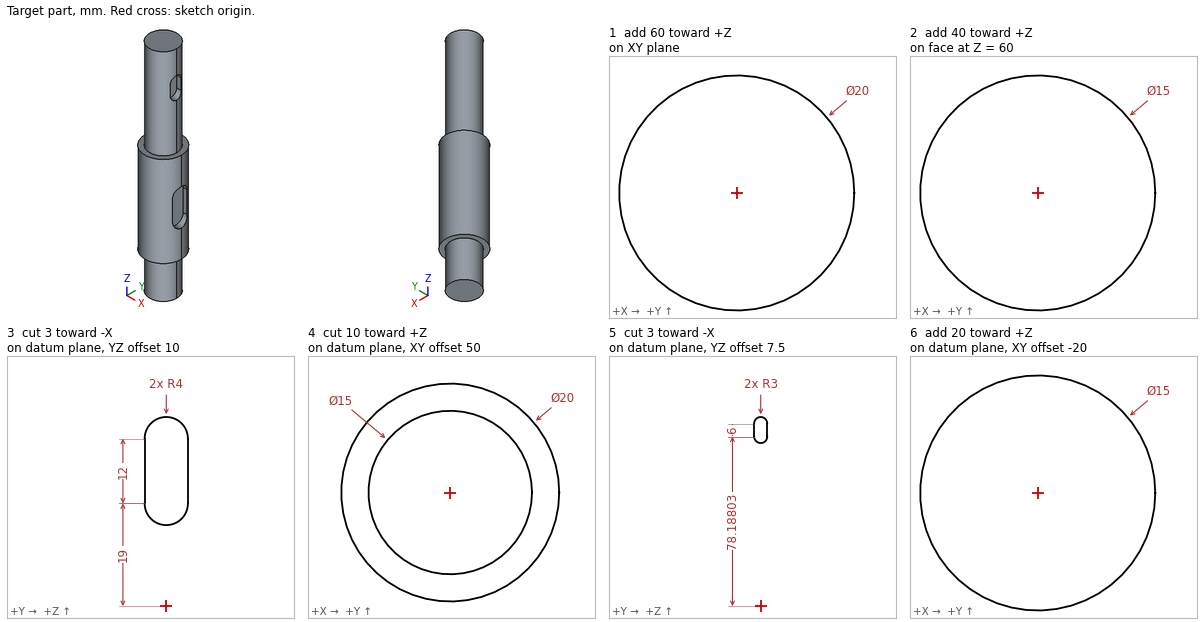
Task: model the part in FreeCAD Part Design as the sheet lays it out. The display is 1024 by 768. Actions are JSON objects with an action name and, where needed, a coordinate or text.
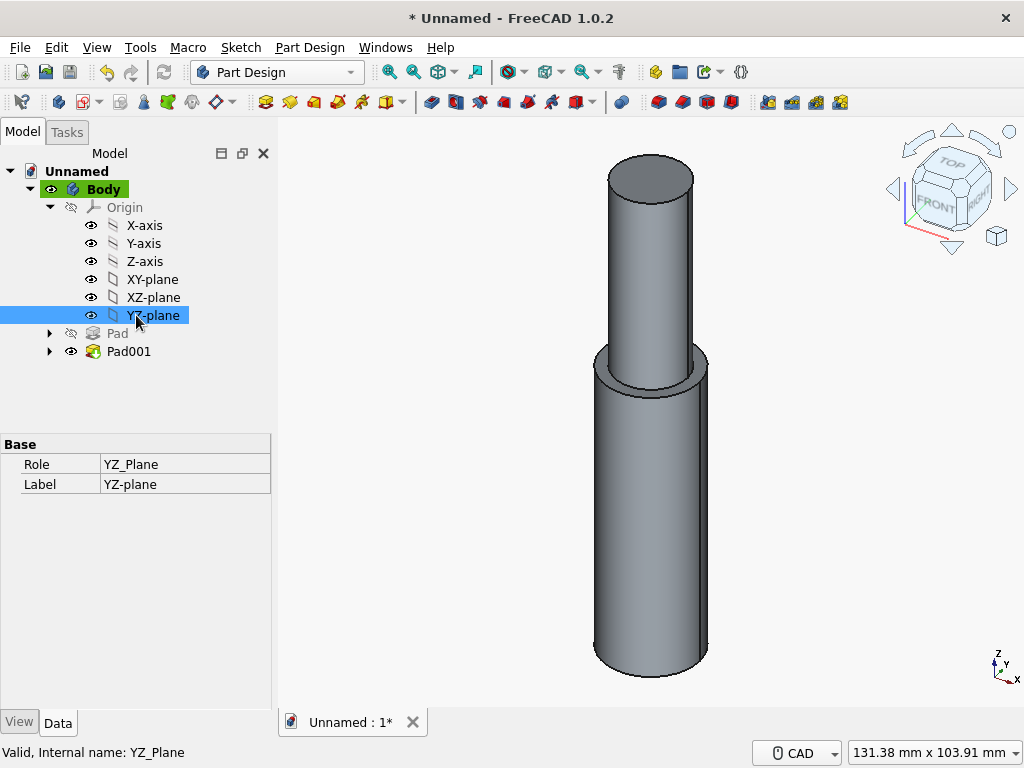
{"action": "left_click", "coordinate": [216, 102]}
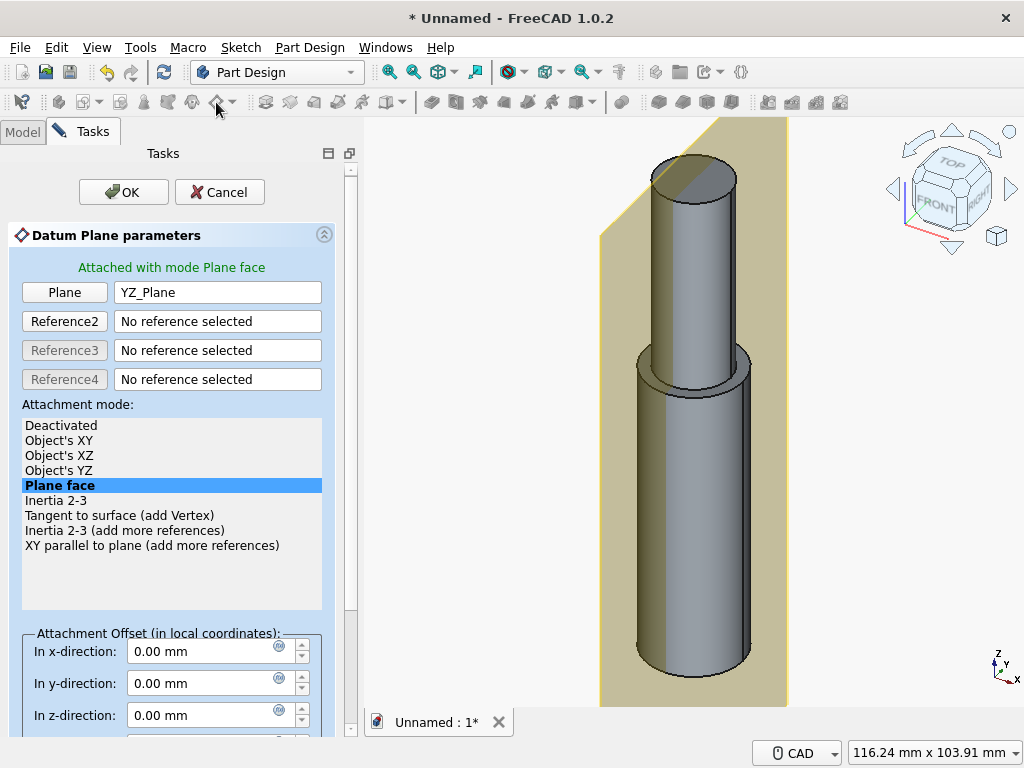
{"action": "triple_click", "coordinate": [210, 715]}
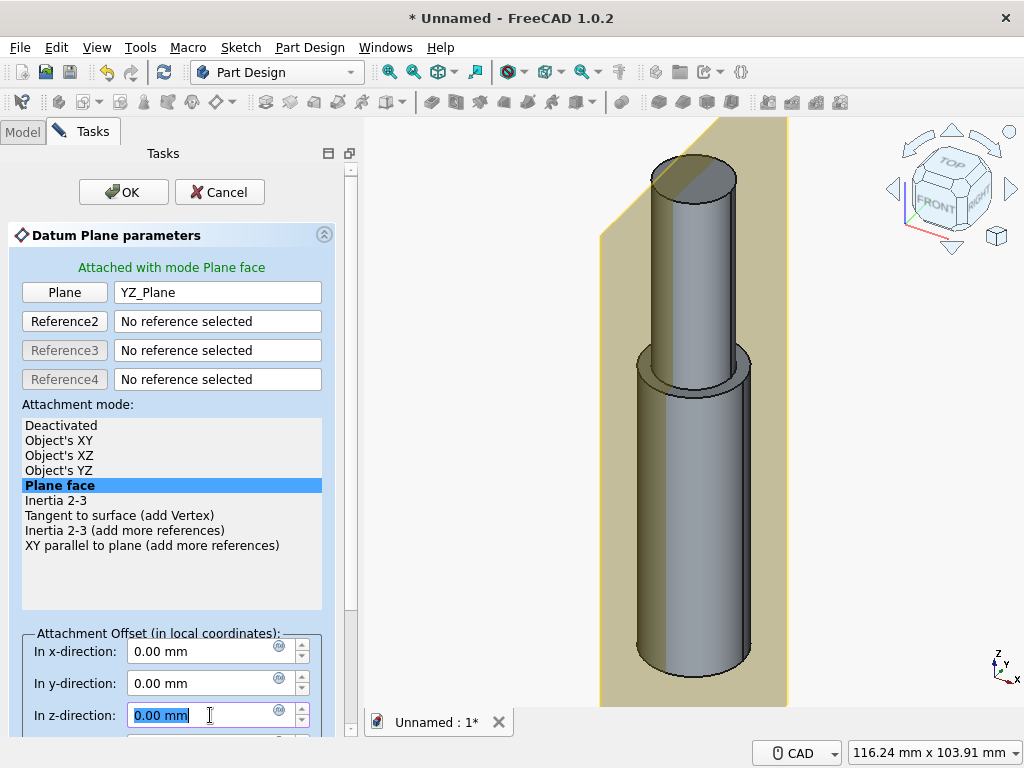
{"action": "type", "text": "10"}
{"action": "key", "text": "Tab"}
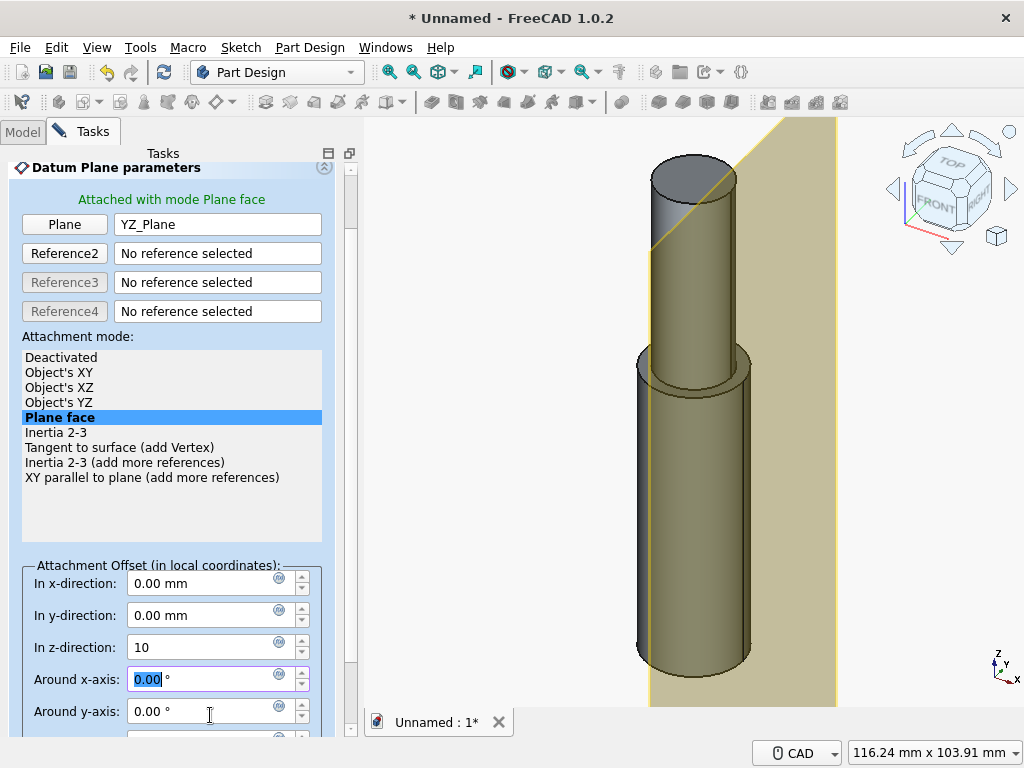
{"action": "scroll", "coordinate": [351, 450], "scroll_direction": "up", "scroll_amount": 2}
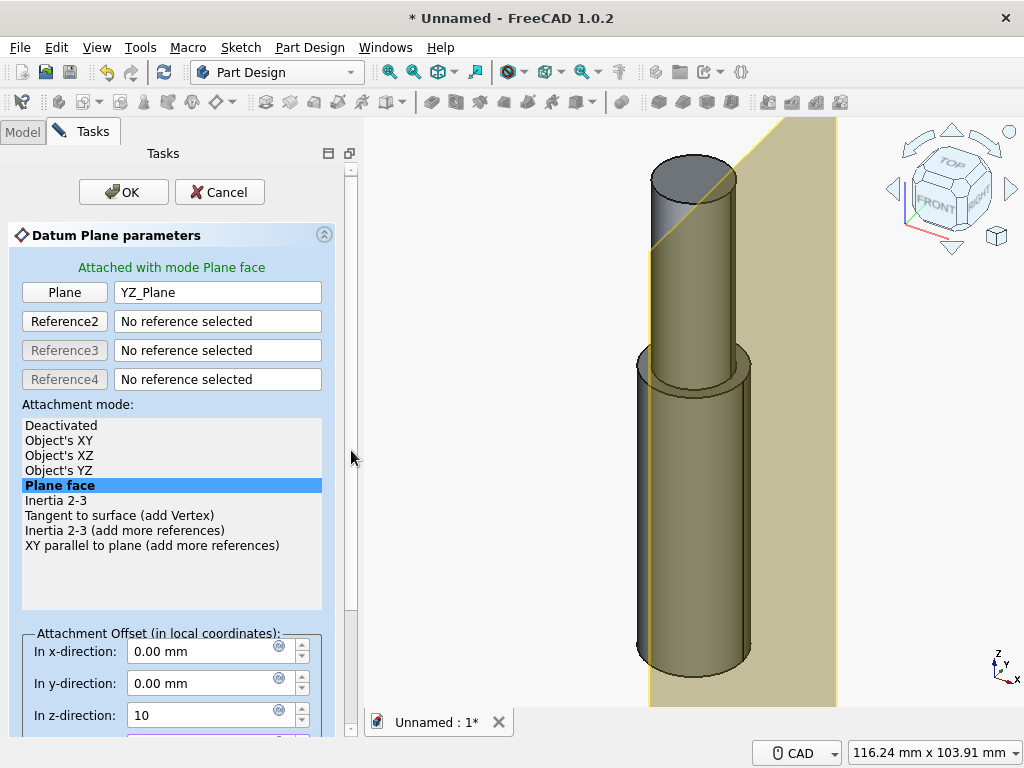
{"action": "left_click", "coordinate": [124, 192]}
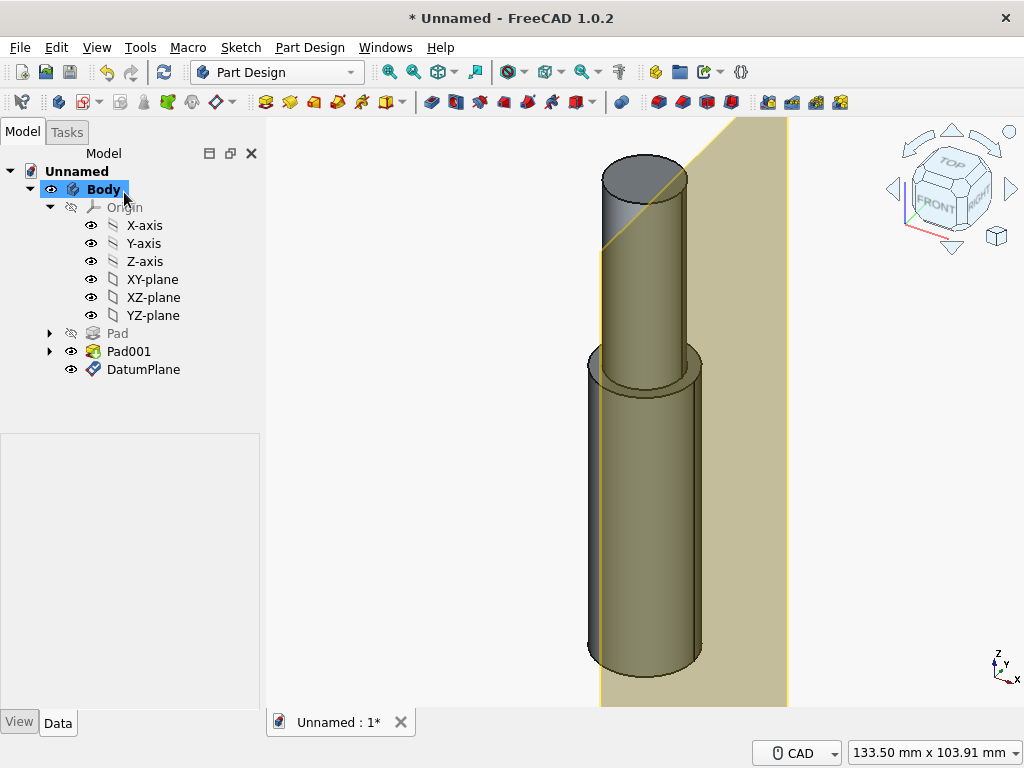
{"action": "left_click", "coordinate": [116, 369]}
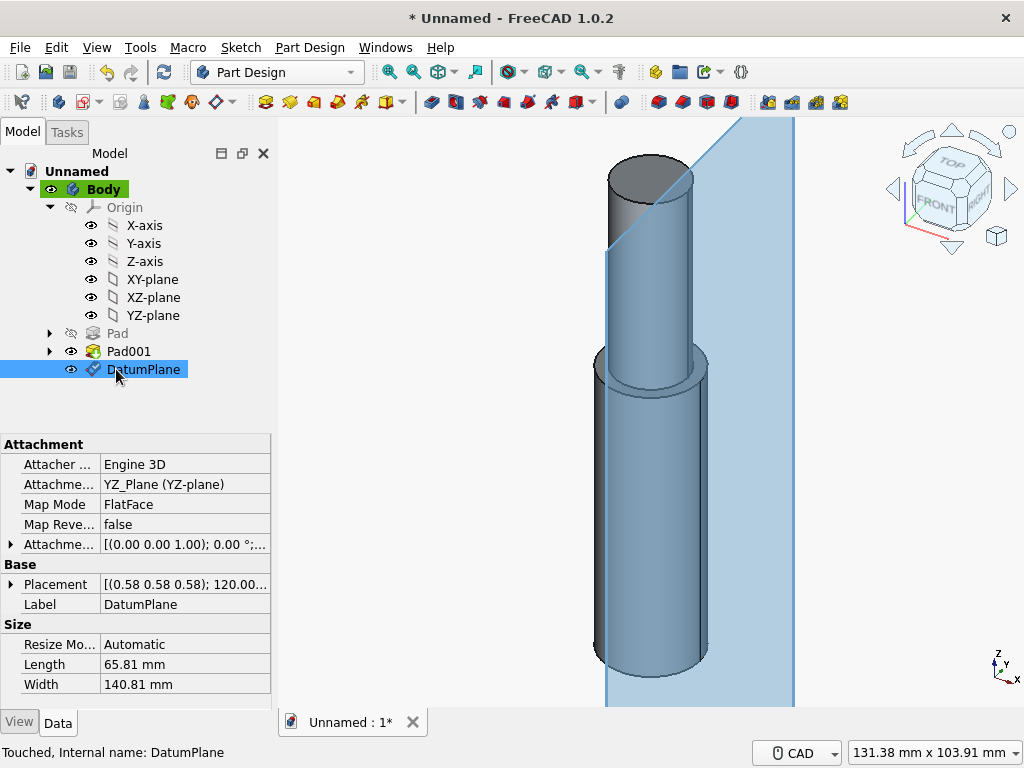
{"action": "left_click", "coordinate": [84, 102]}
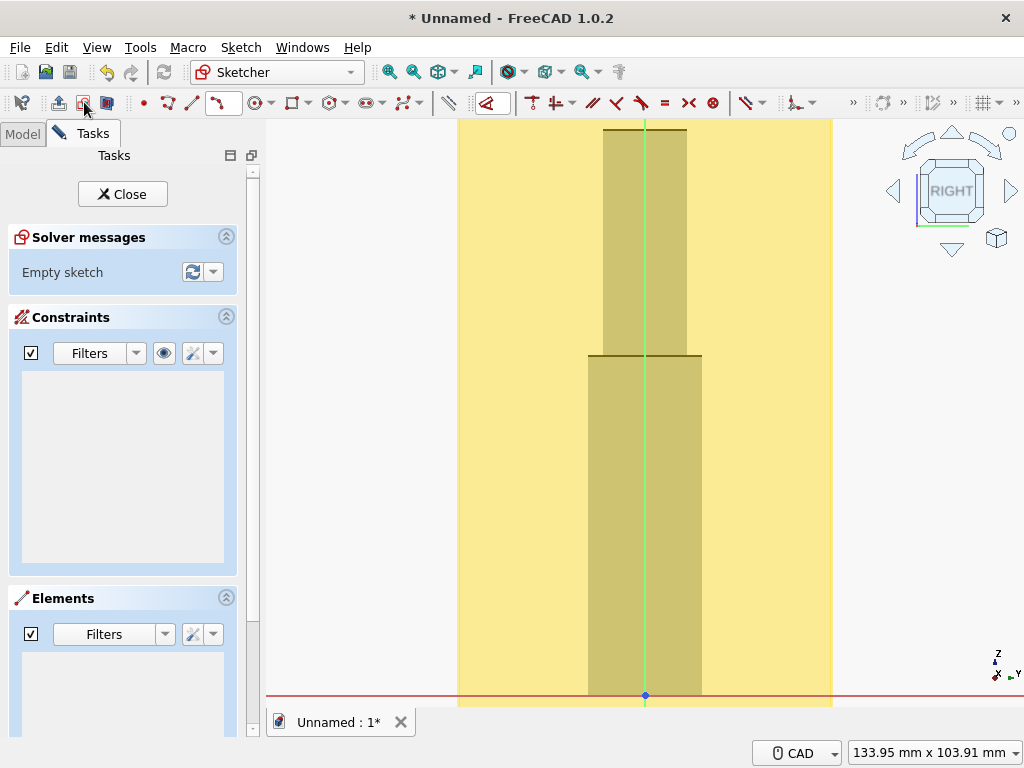
{"action": "scroll", "coordinate": [576, 413], "scroll_direction": "down", "scroll_amount": 5}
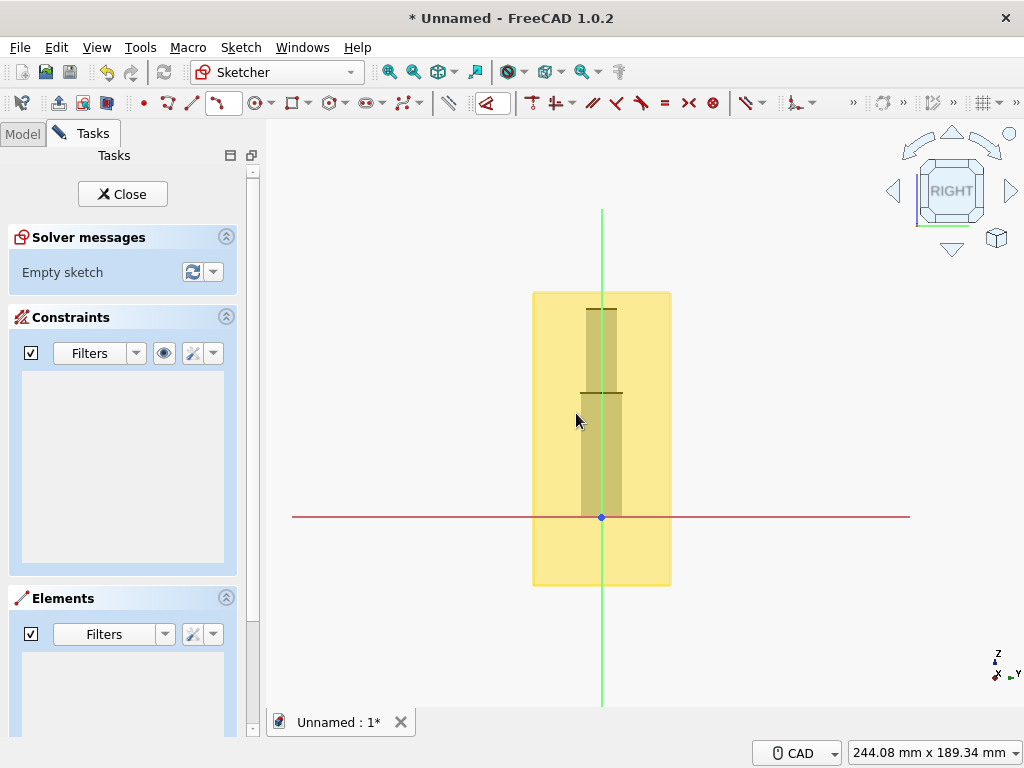
{"action": "scroll", "coordinate": [608, 498], "scroll_direction": "up", "scroll_amount": 8}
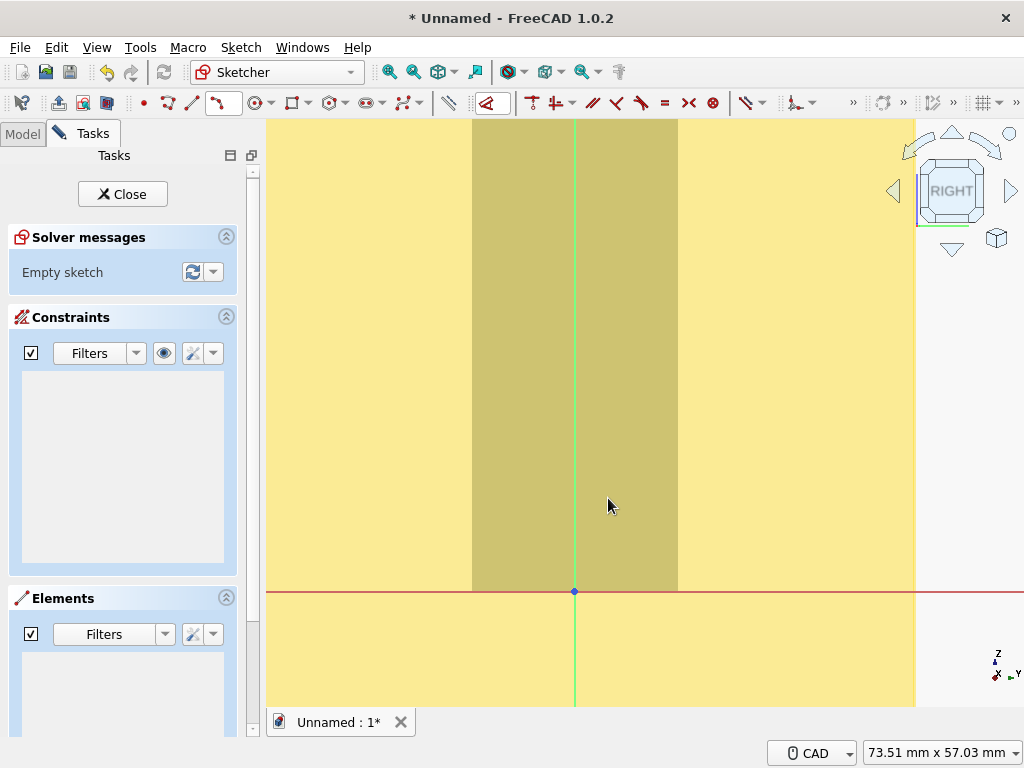
{"action": "left_click", "coordinate": [366, 104]}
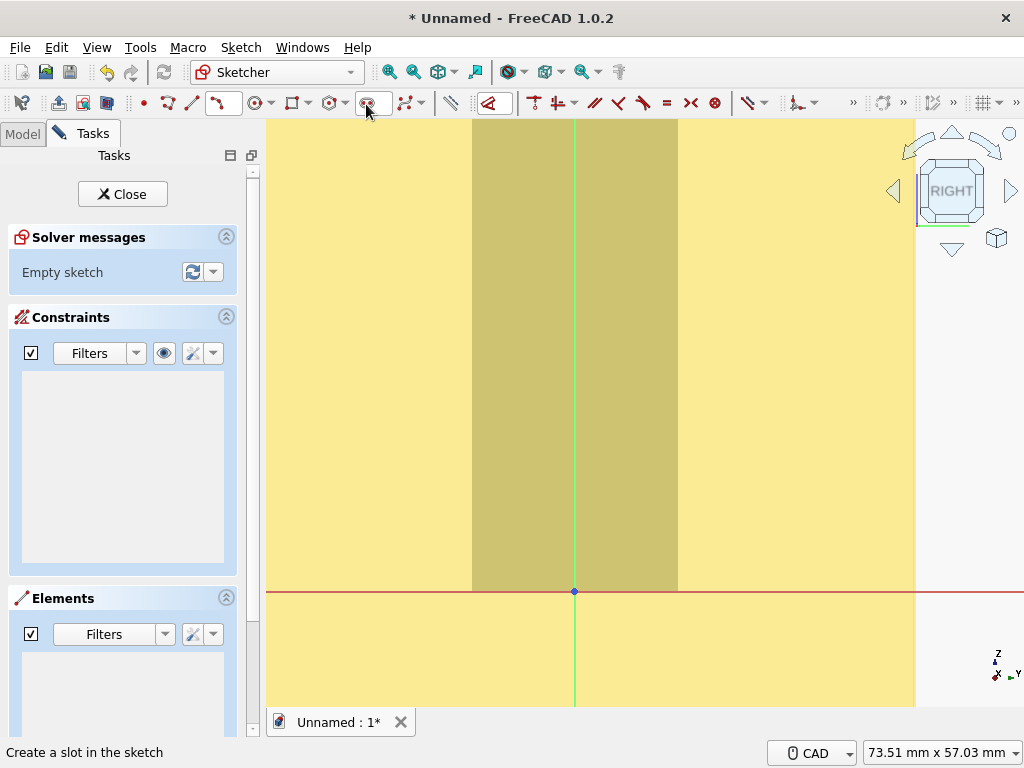
{"action": "left_click", "coordinate": [575, 396]}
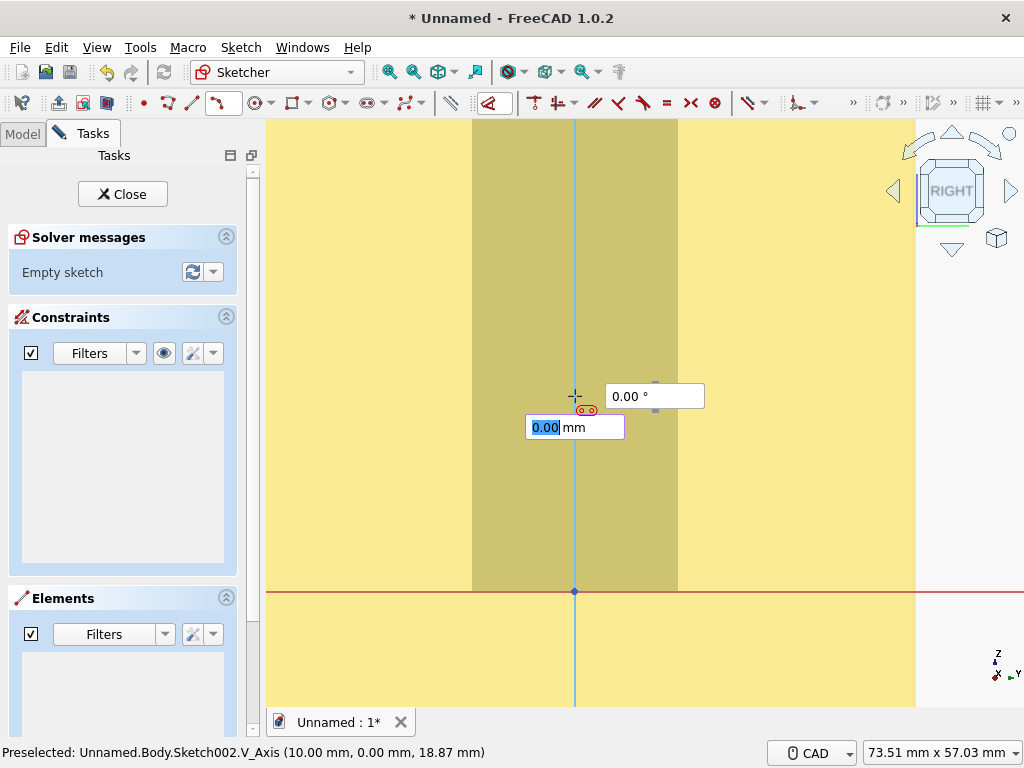
{"action": "left_click", "coordinate": [584, 272]}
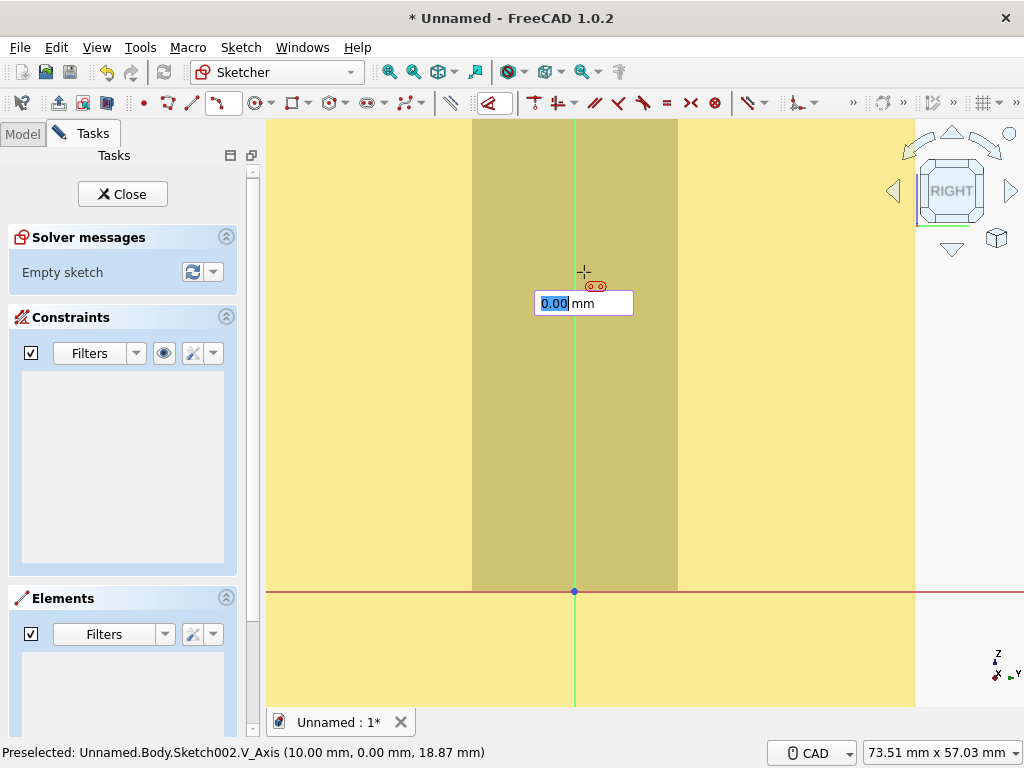
{"action": "left_click", "coordinate": [616, 334]}
{"action": "key", "text": "Escape"}